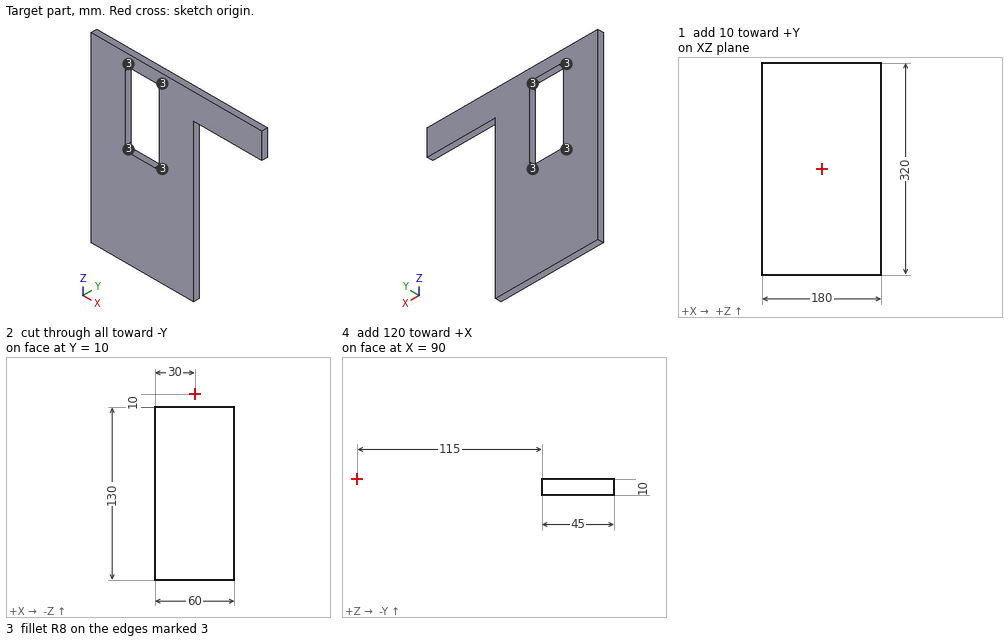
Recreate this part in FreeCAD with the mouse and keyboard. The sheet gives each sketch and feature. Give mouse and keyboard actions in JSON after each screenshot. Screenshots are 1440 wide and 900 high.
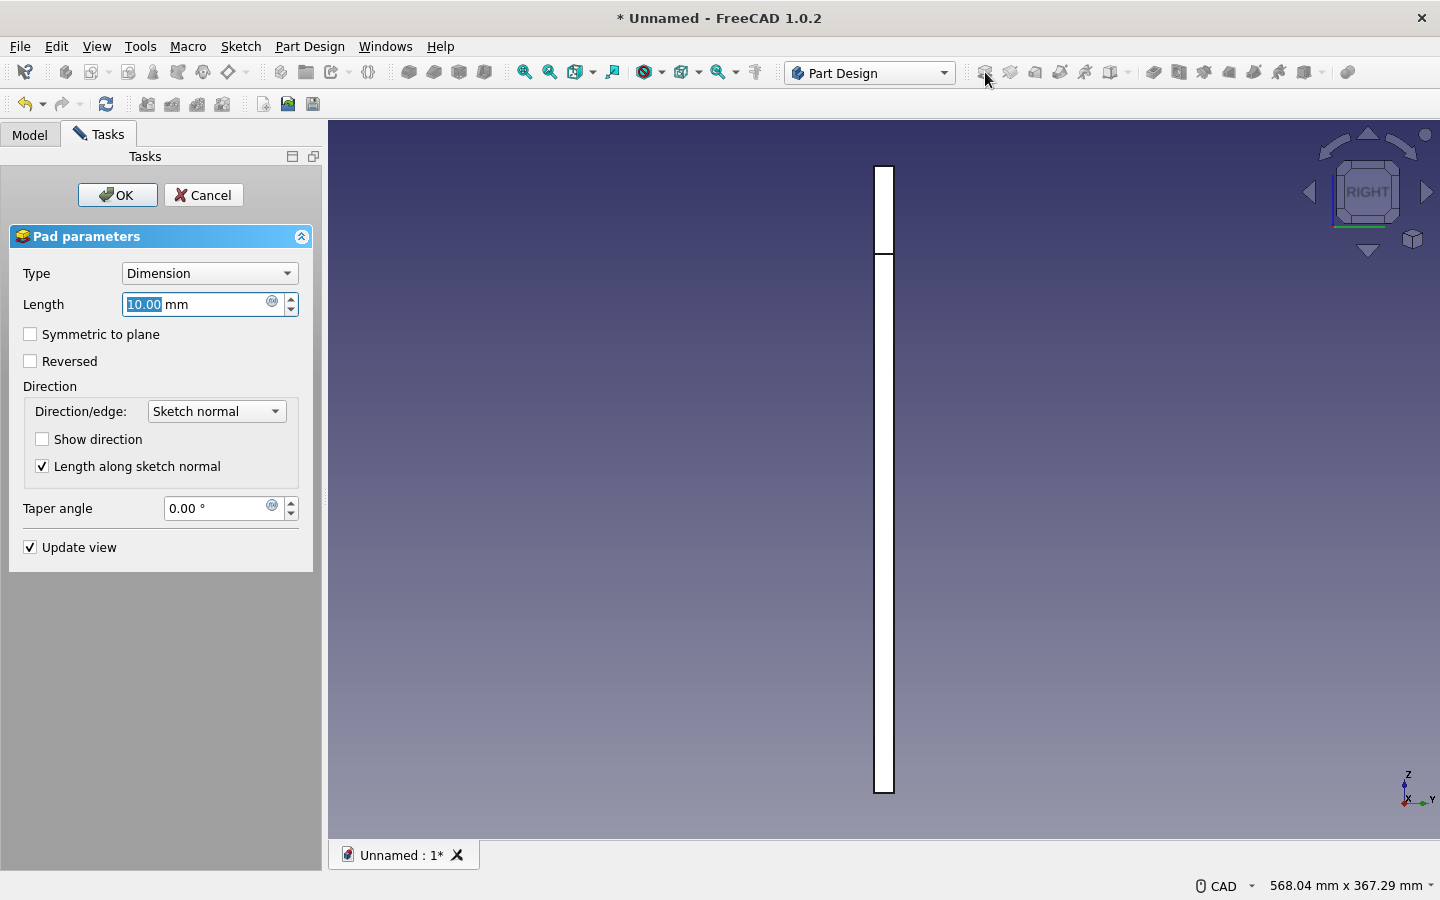
{"action": "type", "text": "120"}
{"action": "key", "text": "Tab"}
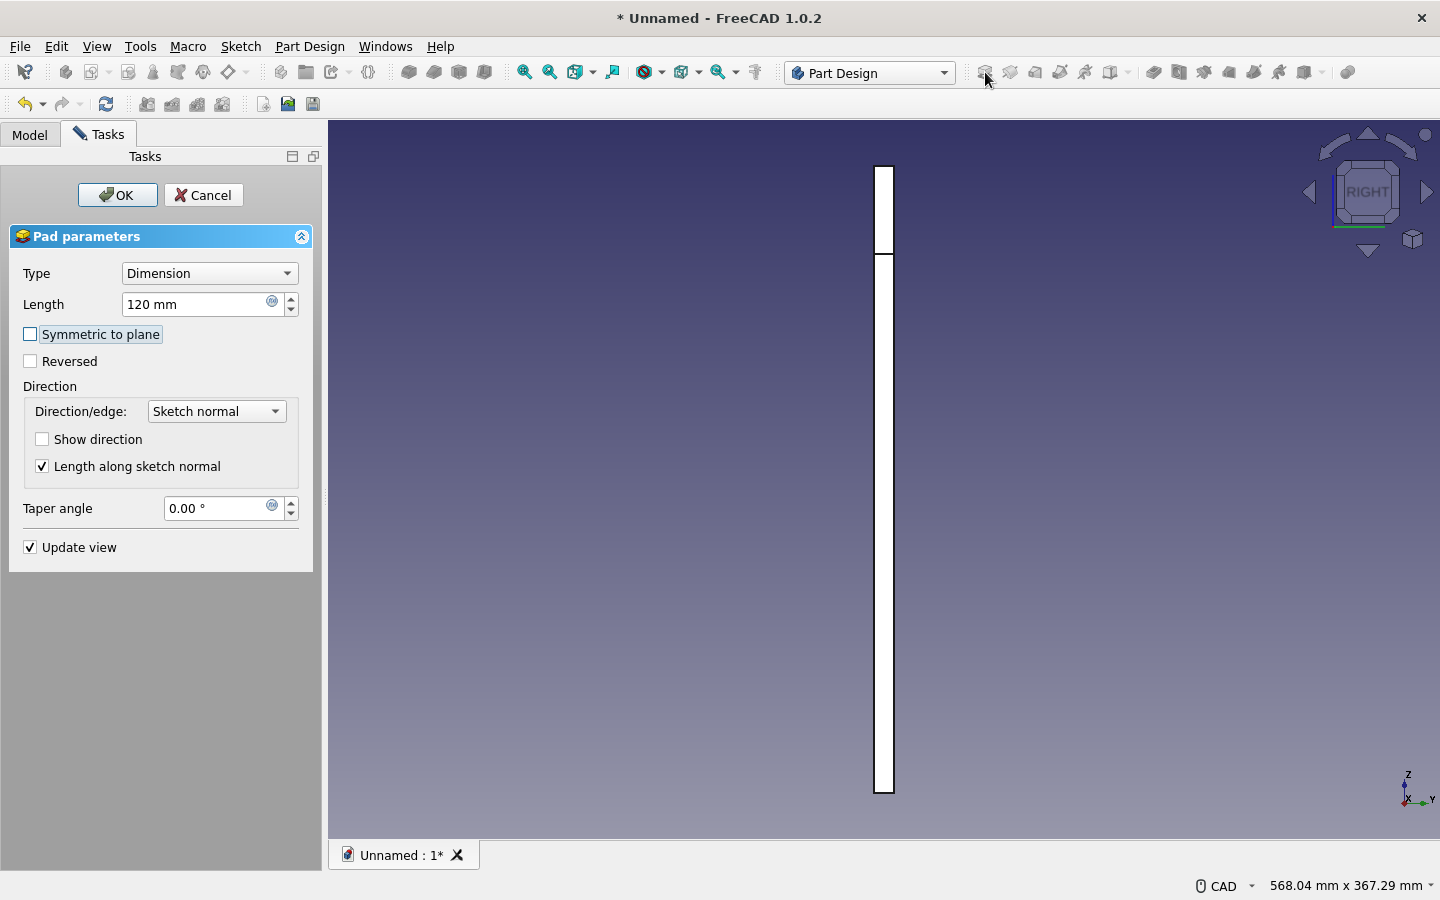
{"action": "left_click", "coordinate": [118, 195]}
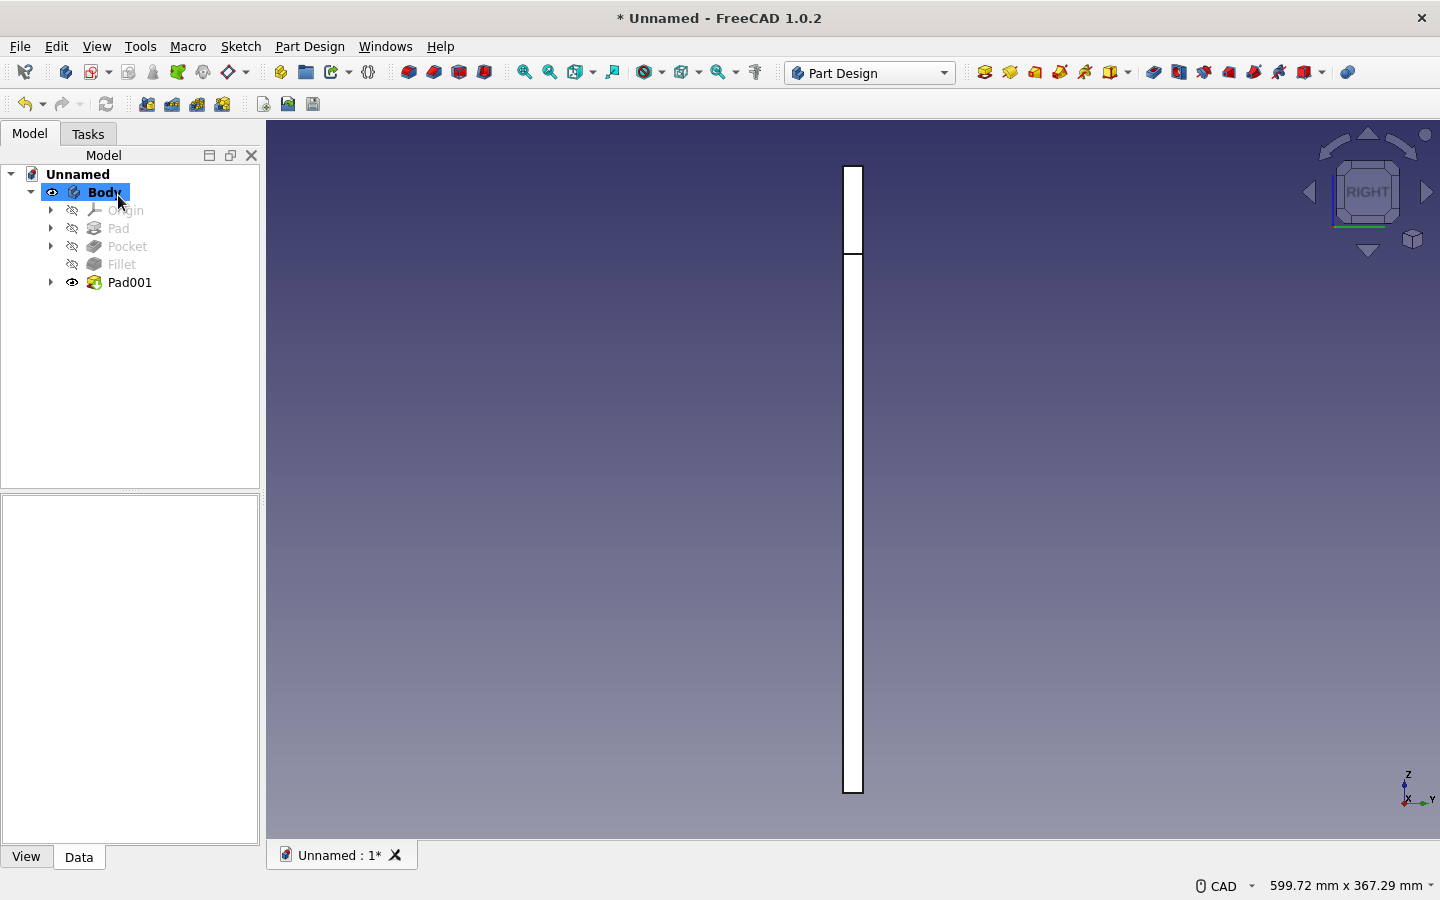
{"action": "key", "text": "0"}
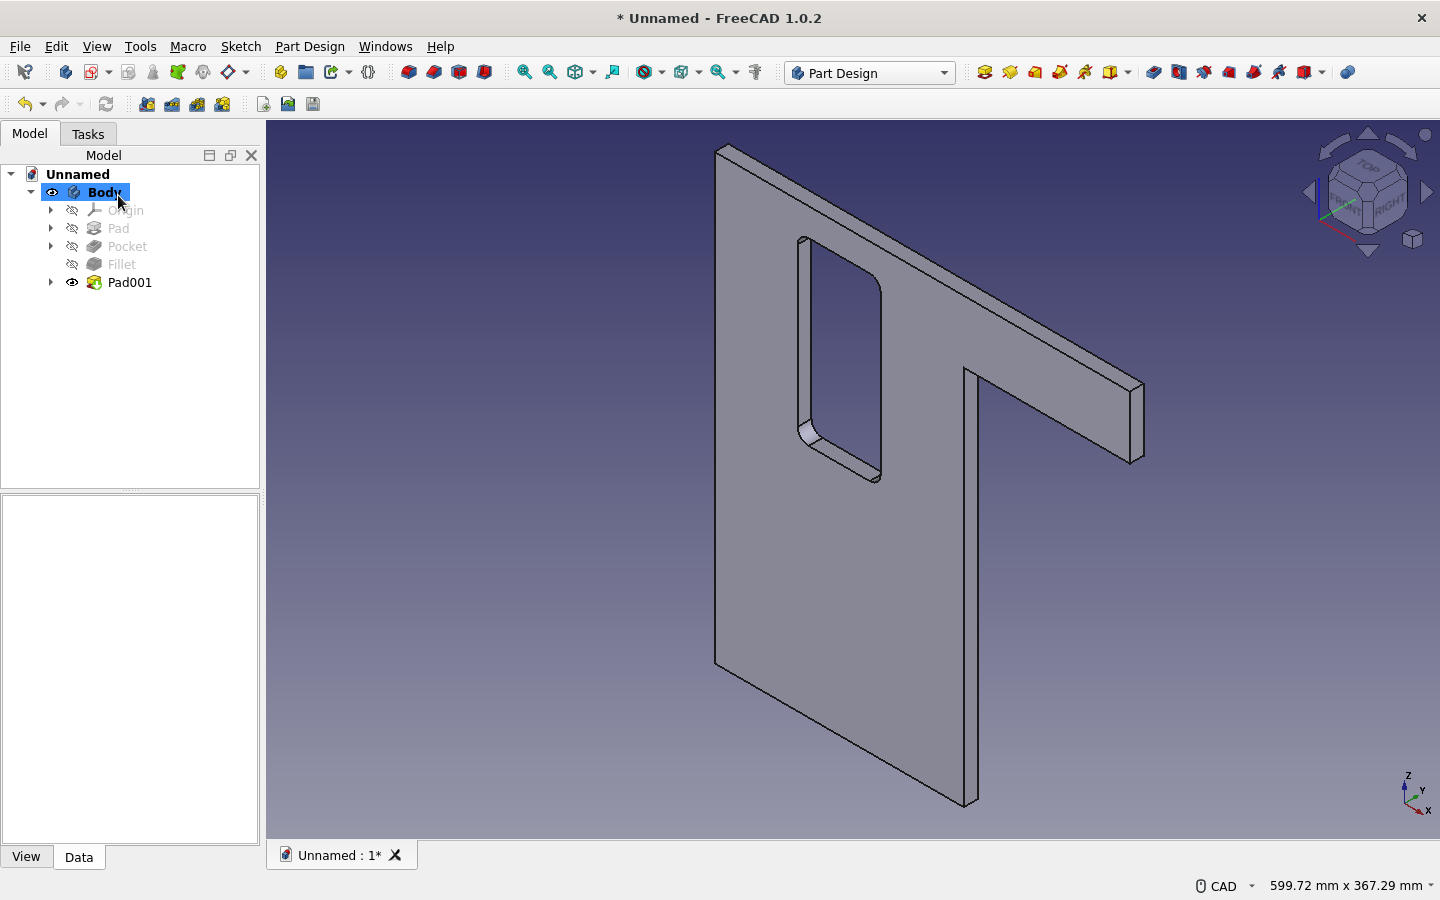
{"action": "left_click", "coordinate": [525, 72]}